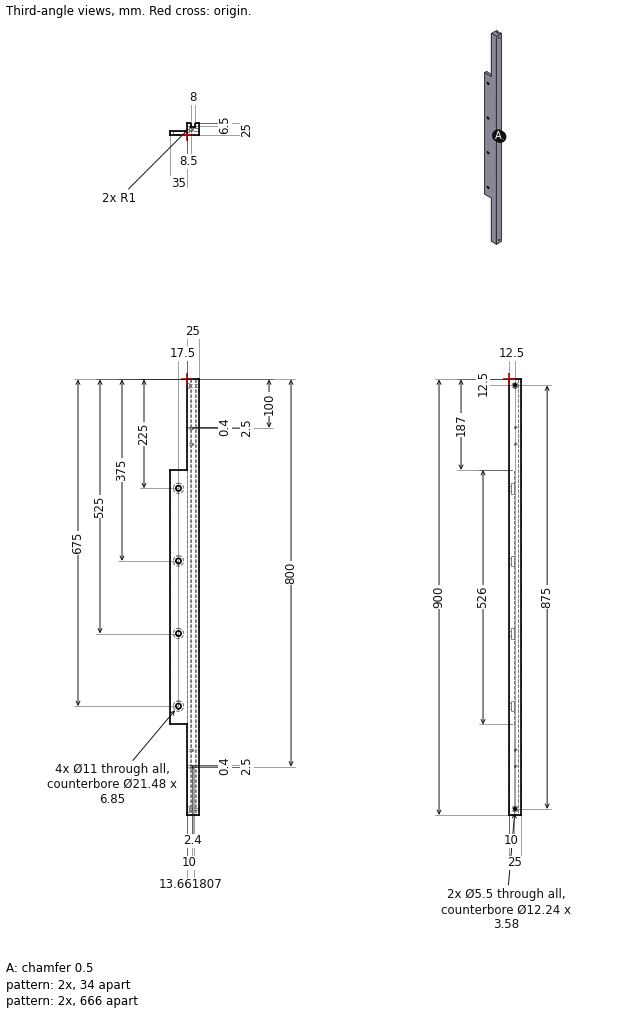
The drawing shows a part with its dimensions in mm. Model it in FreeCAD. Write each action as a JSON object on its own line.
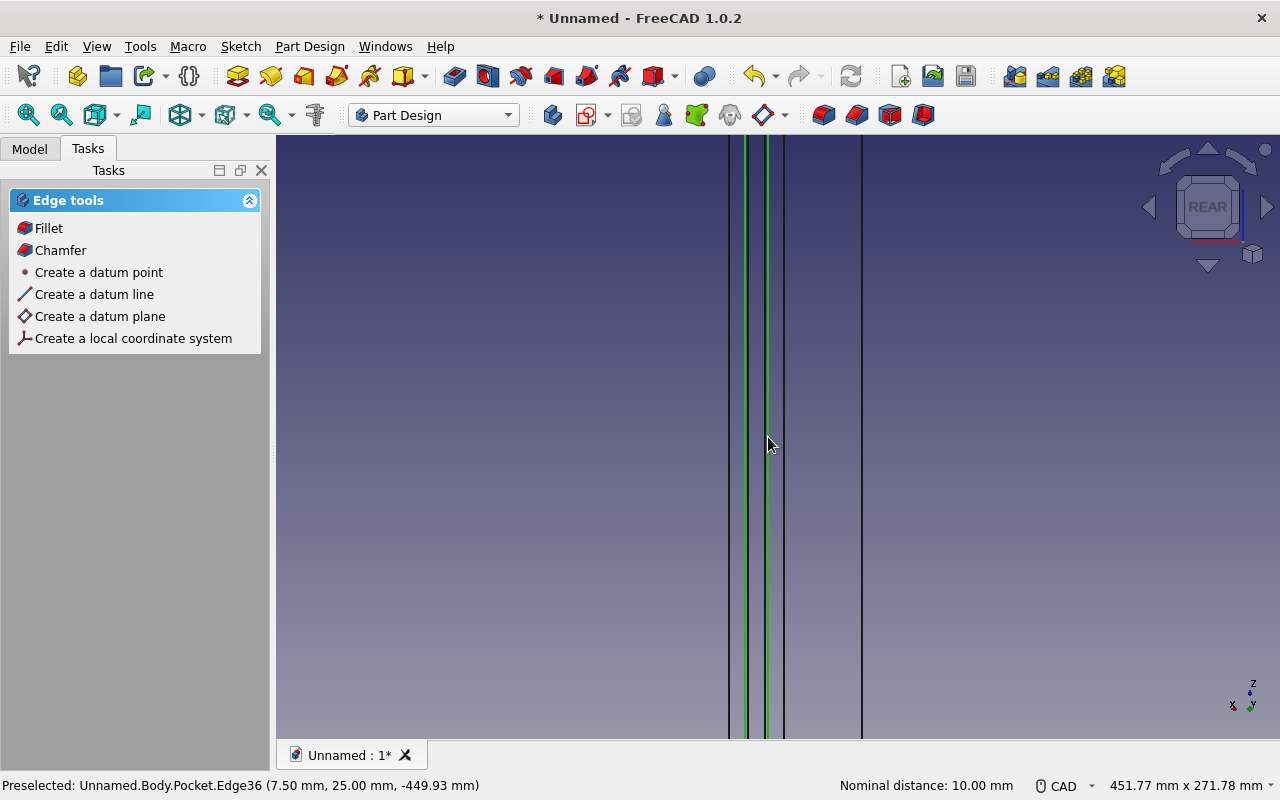
{"action": "key", "text": "v 1"}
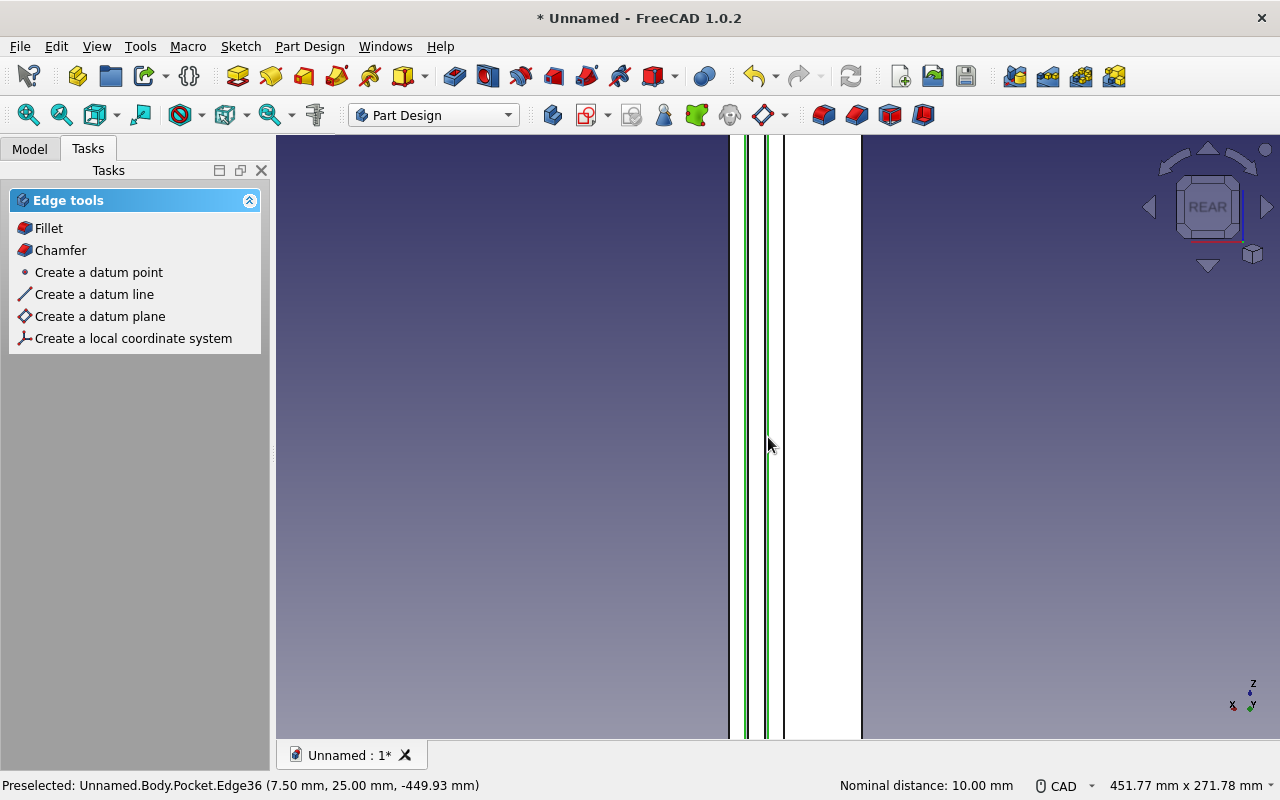
{"action": "left_click", "coordinate": [857, 116]}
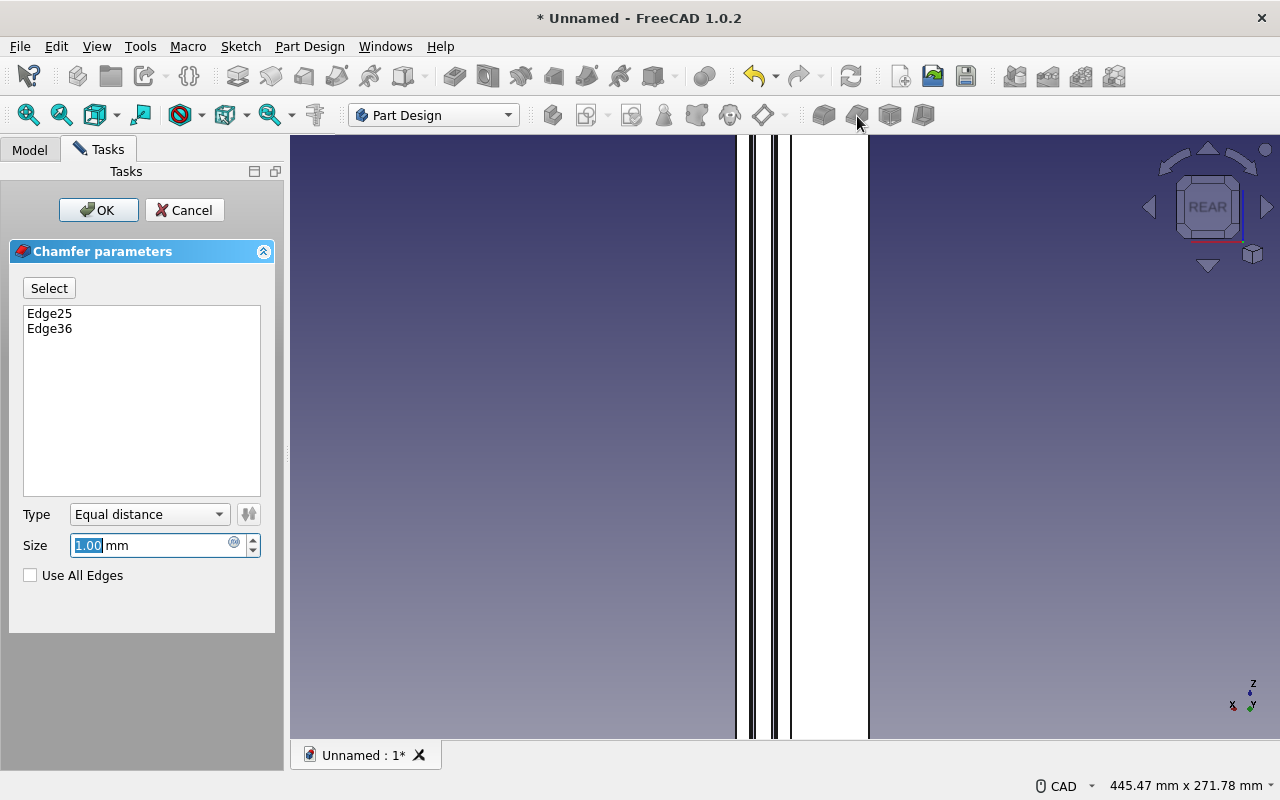
{"action": "type", "text": "0.5"}
{"action": "key", "text": "Tab"}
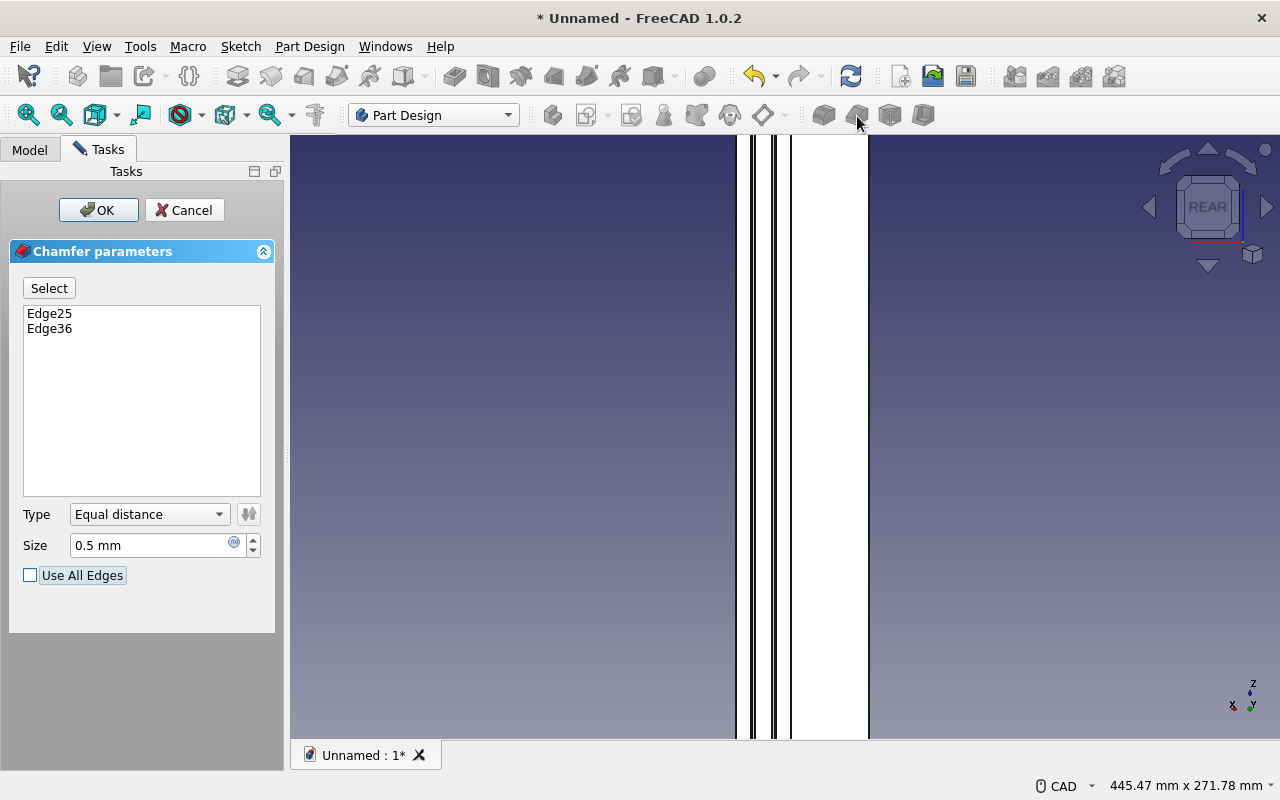
{"action": "left_click", "coordinate": [99, 210]}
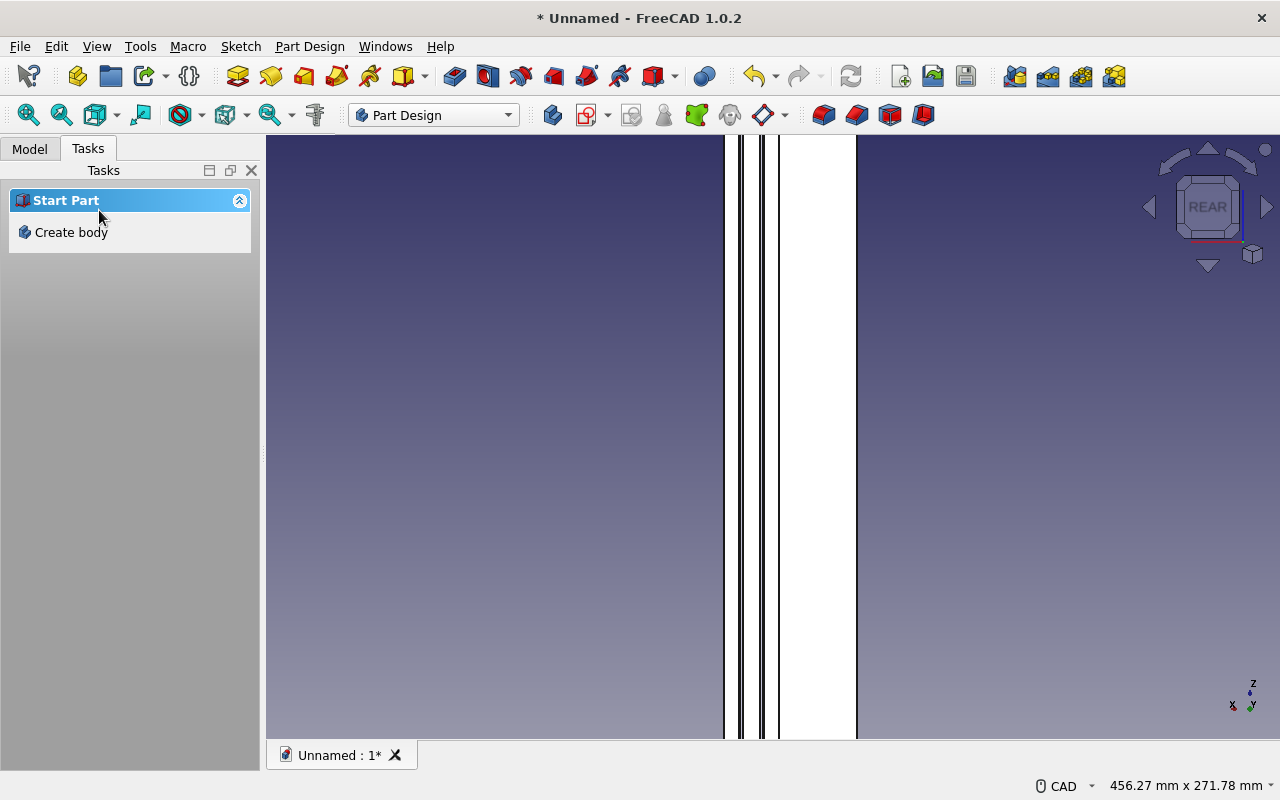
{"action": "left_click", "coordinate": [29, 116]}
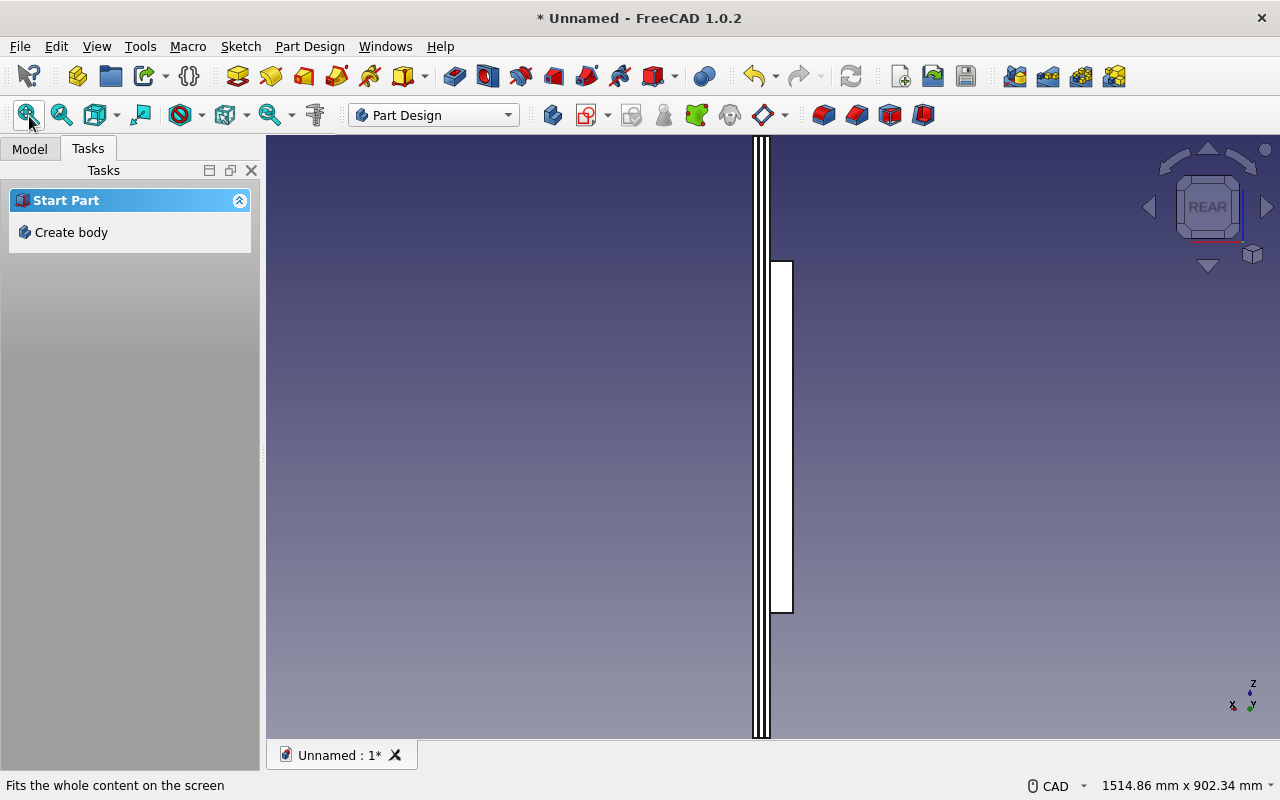
{"action": "left_click", "coordinate": [781, 587]}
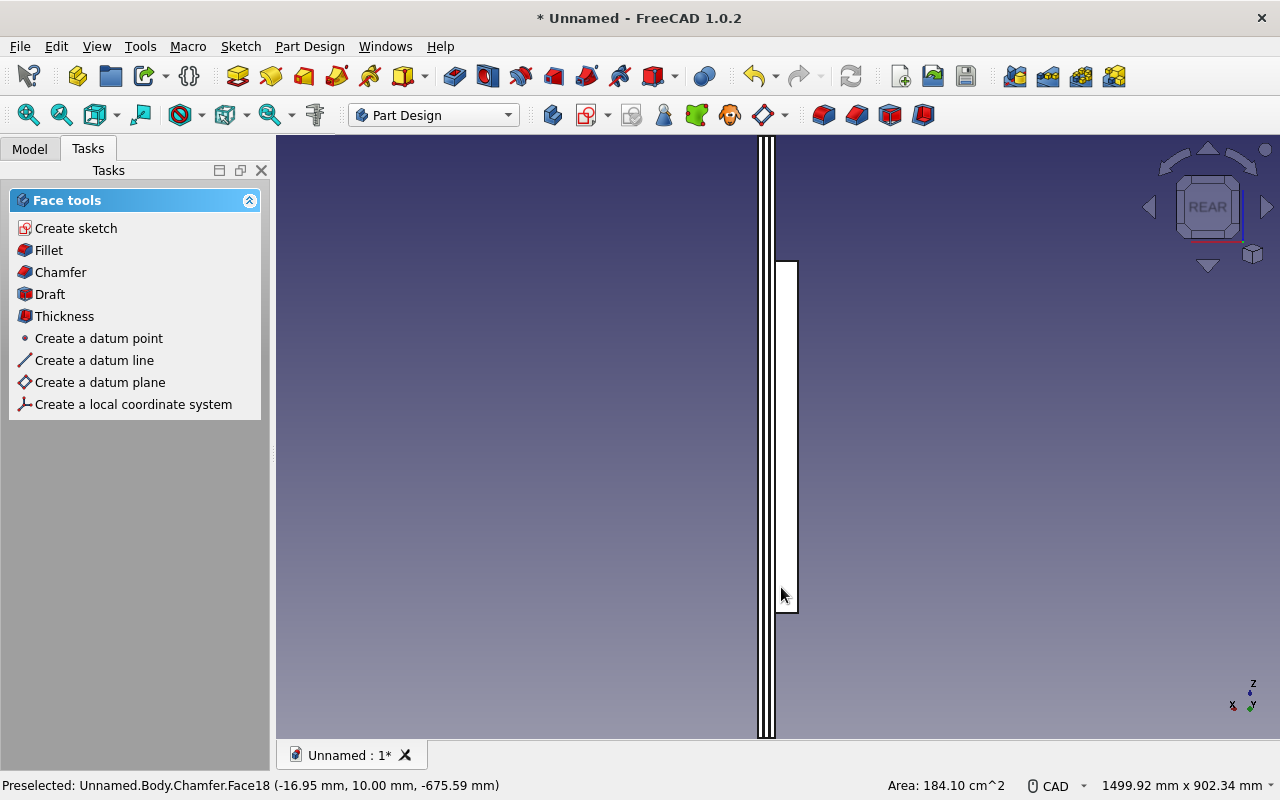
{"action": "left_click", "coordinate": [586, 116]}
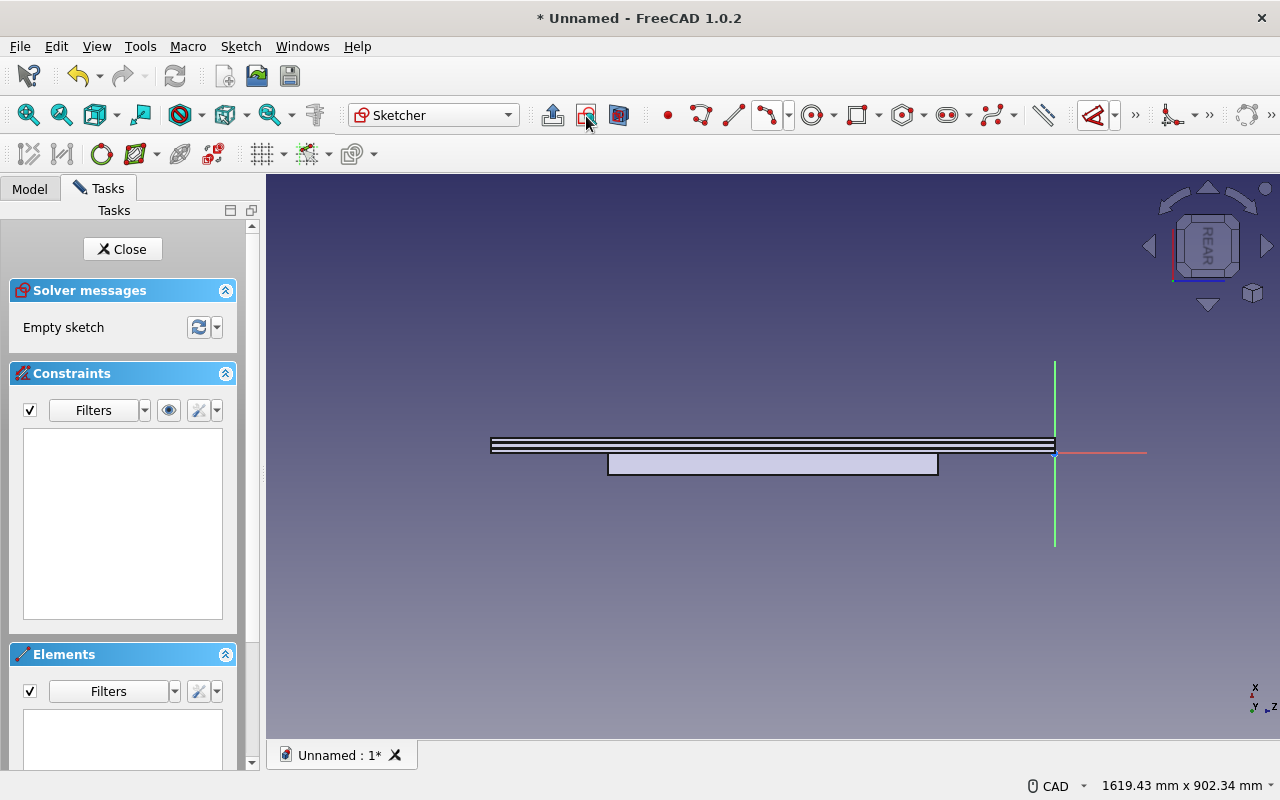
{"action": "left_click", "coordinate": [619, 116]}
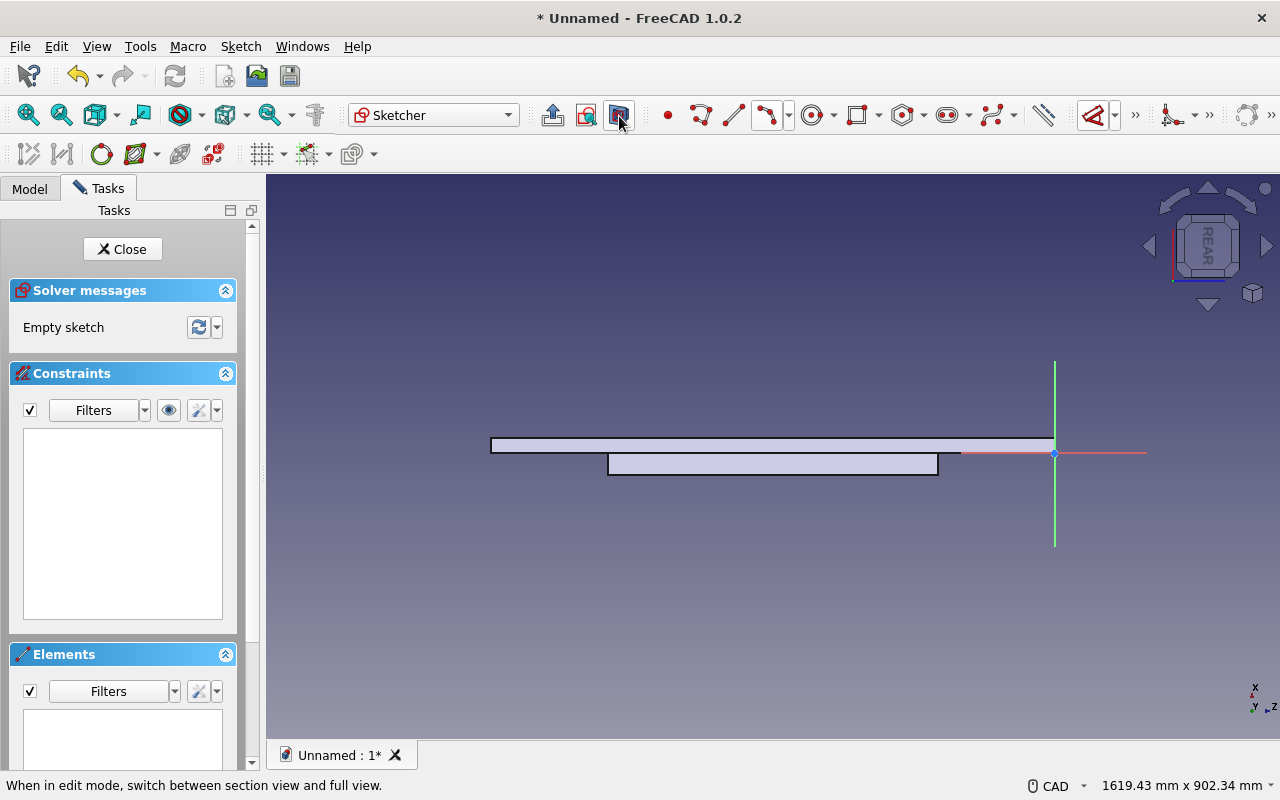
{"action": "scroll", "coordinate": [1115, 469], "scroll_direction": "up", "scroll_amount": 2}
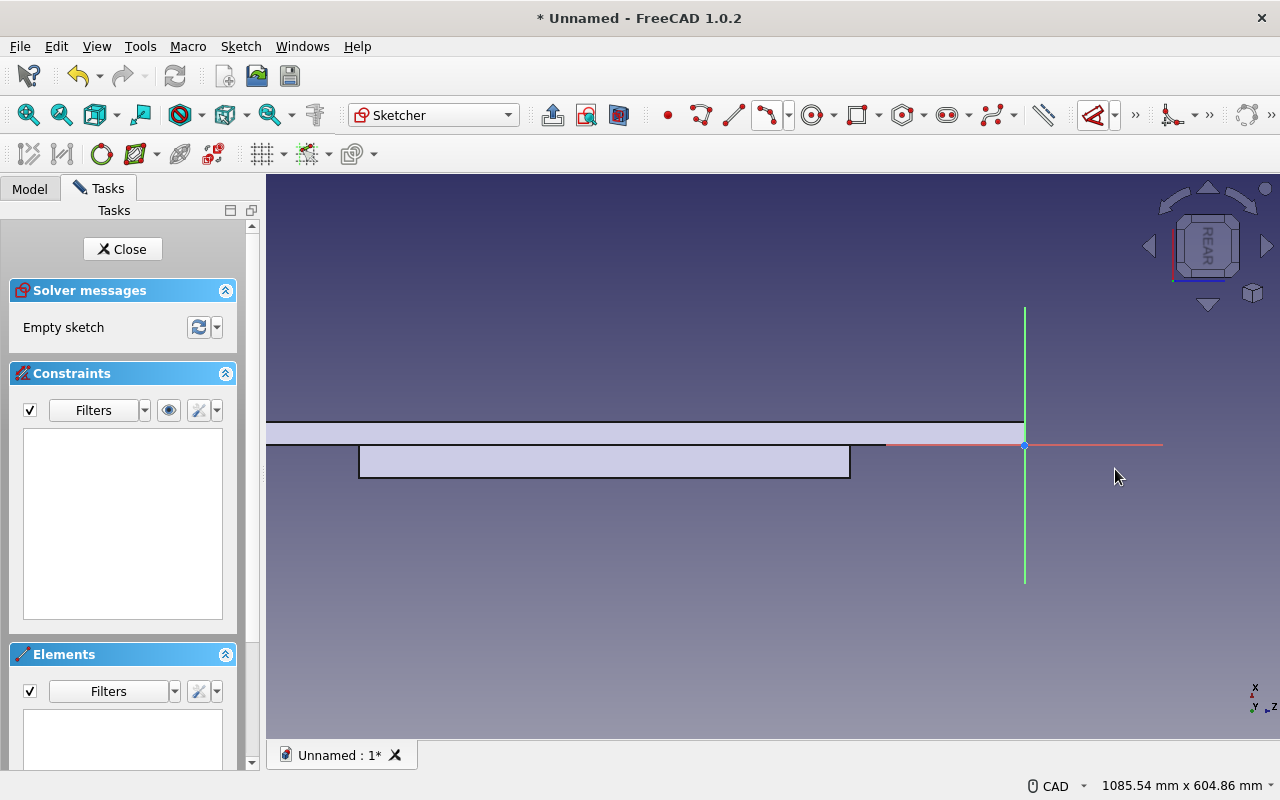
{"action": "left_click", "coordinate": [812, 116]}